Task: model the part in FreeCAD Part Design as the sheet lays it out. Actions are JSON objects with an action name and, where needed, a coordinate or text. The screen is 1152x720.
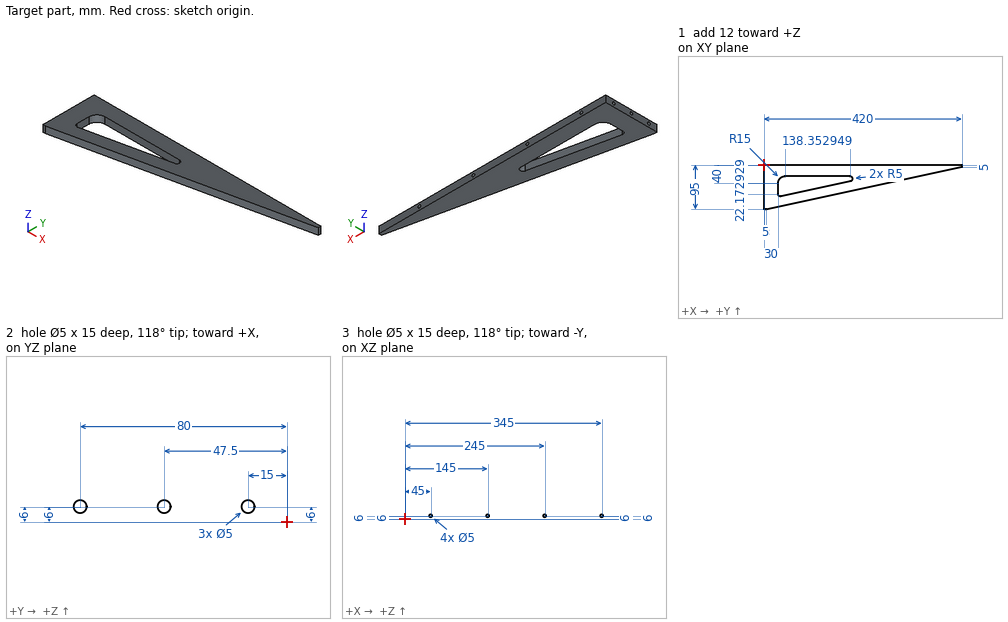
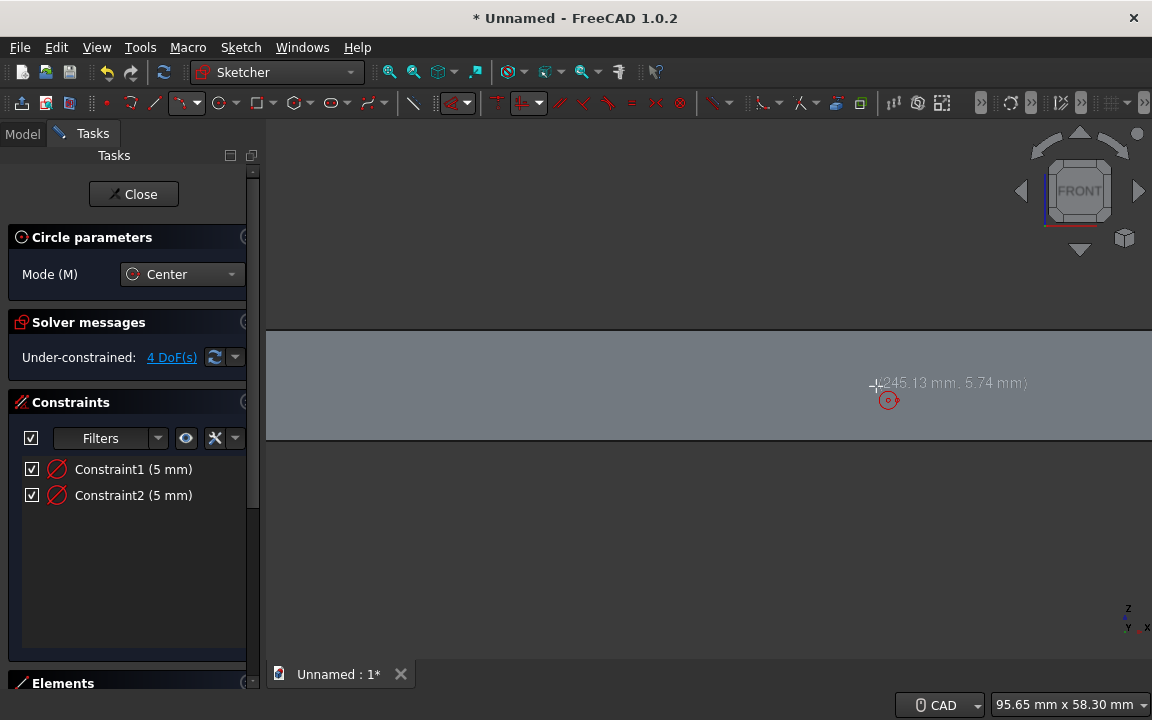
{"action": "scroll", "coordinate": [725, 386], "scroll_direction": "down", "scroll_amount": 9}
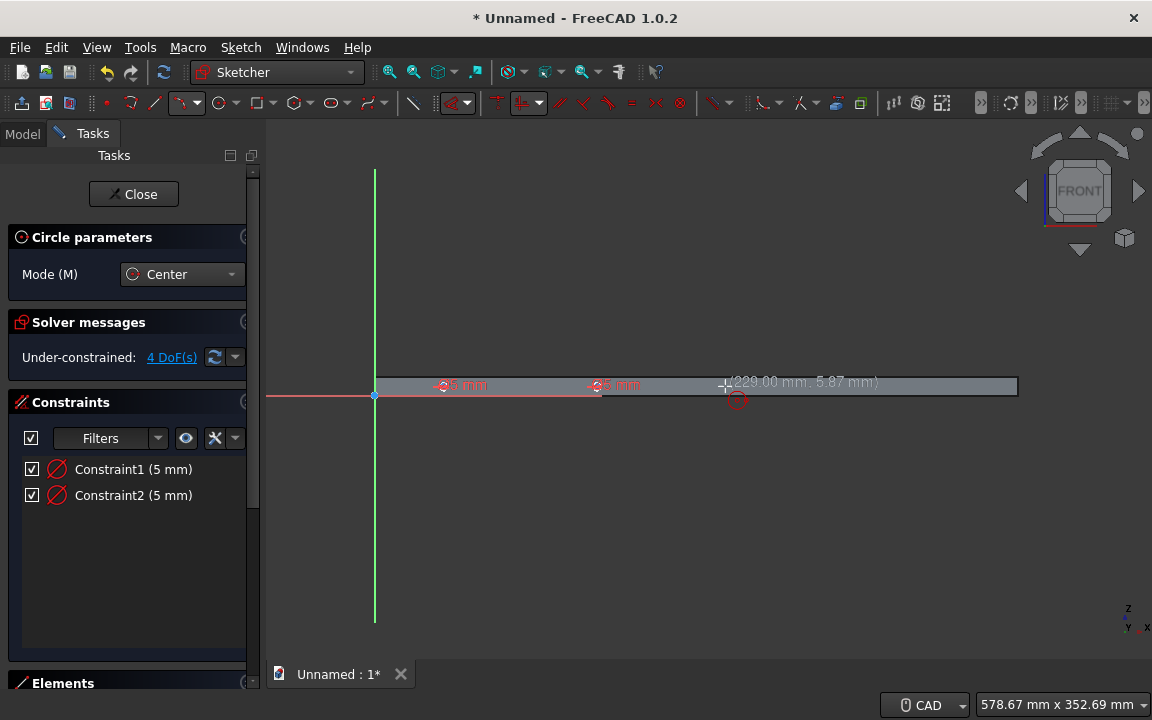
{"action": "scroll", "coordinate": [750, 386], "scroll_direction": "up", "scroll_amount": 3}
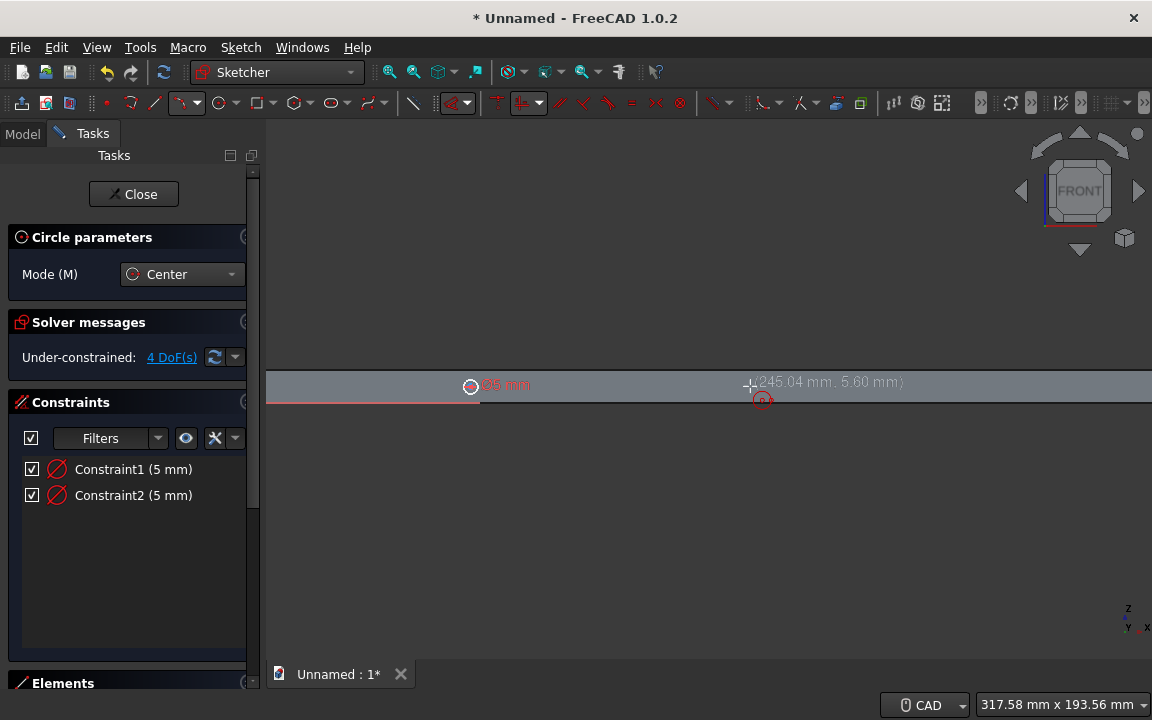
{"action": "left_click", "coordinate": [749, 386]}
{"action": "mouse_move", "coordinate": [754, 381]}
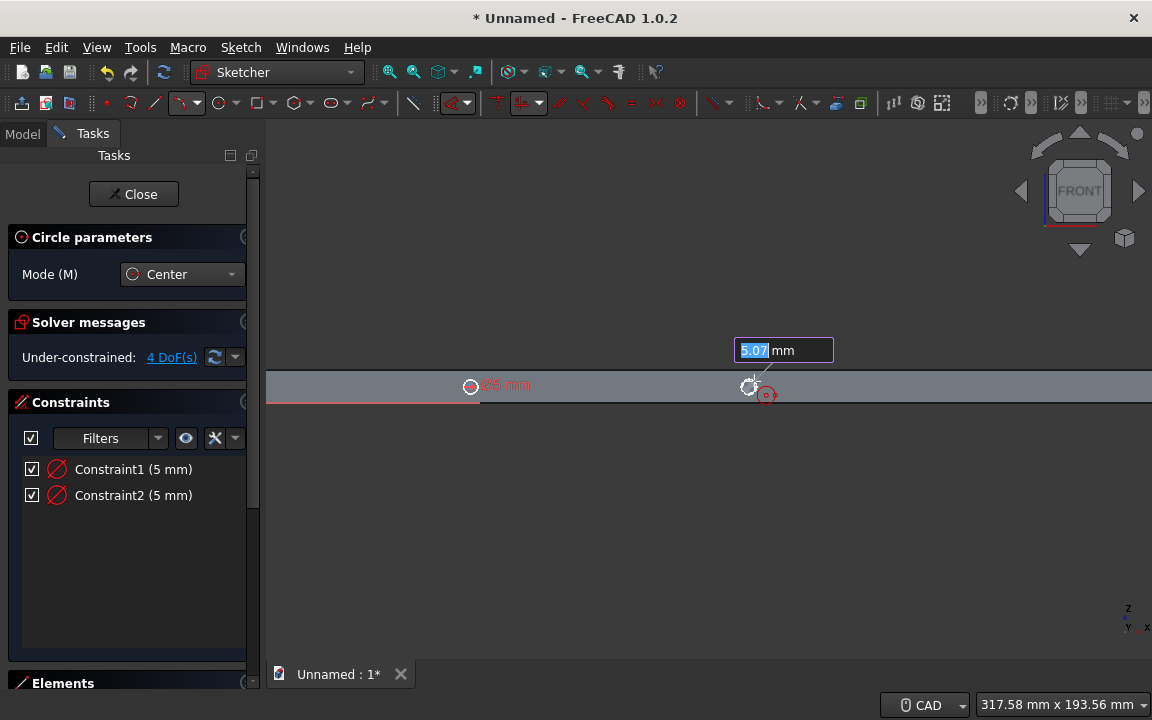
{"action": "type", "text": "5"}
{"action": "key", "text": "Return"}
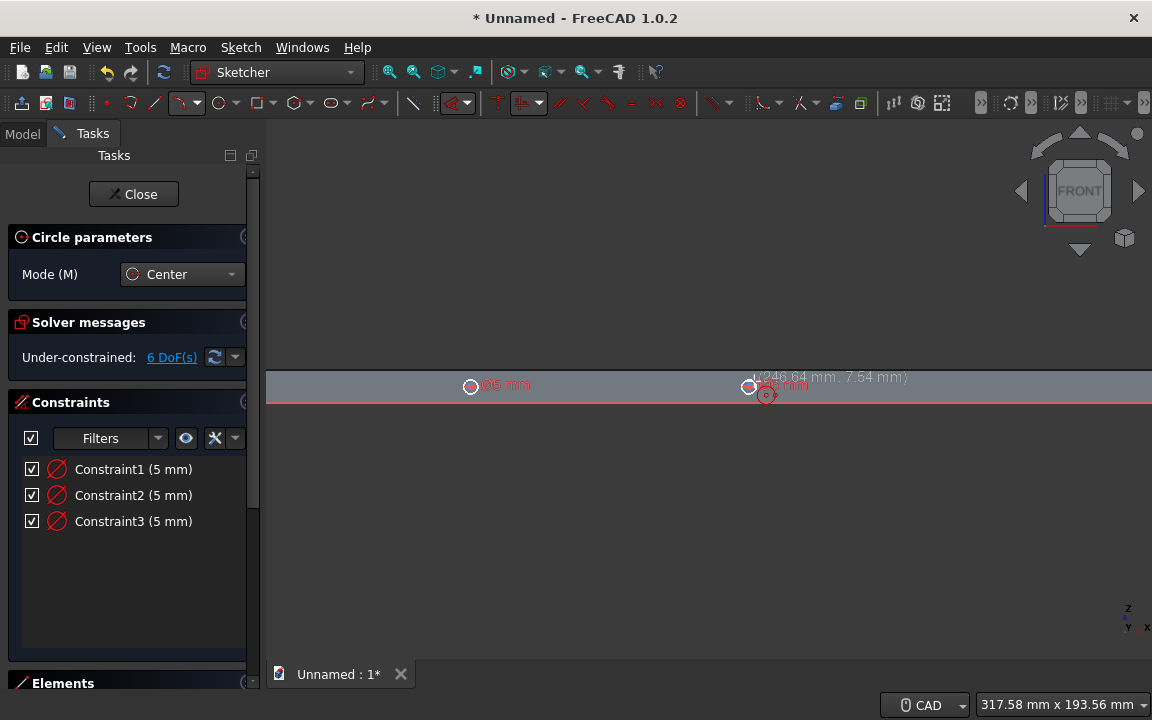
{"action": "scroll", "coordinate": [750, 386], "scroll_direction": "down", "scroll_amount": 3}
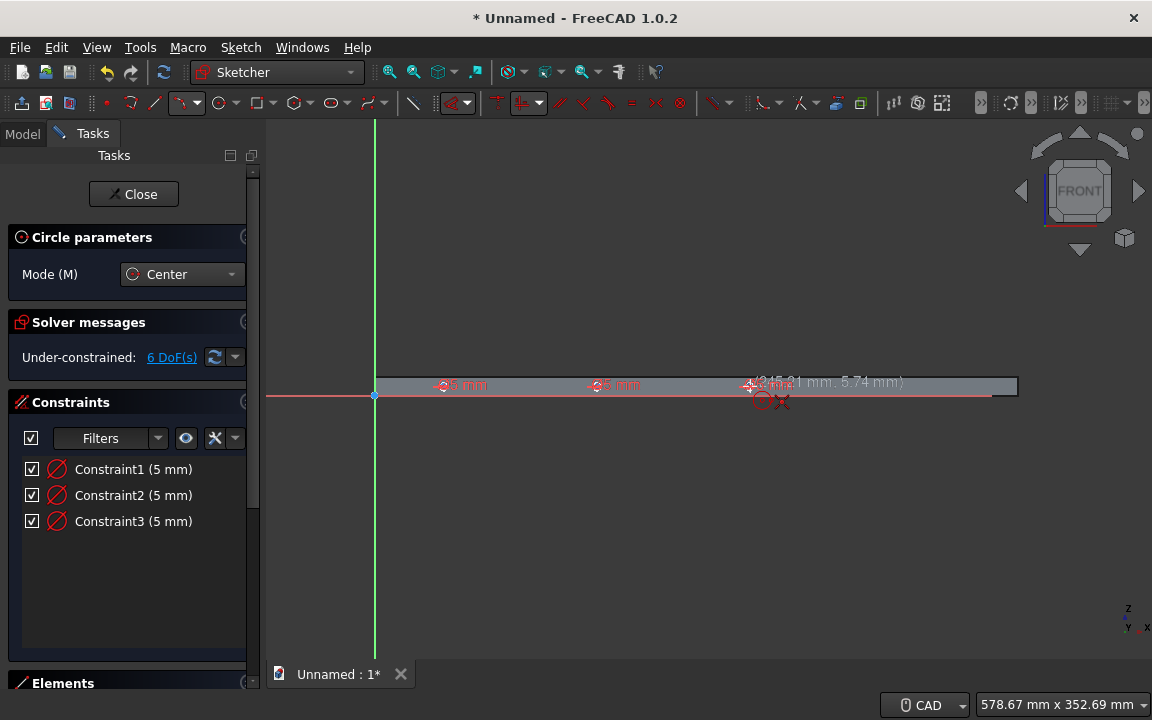
{"action": "scroll", "coordinate": [903, 386], "scroll_direction": "up", "scroll_amount": 9}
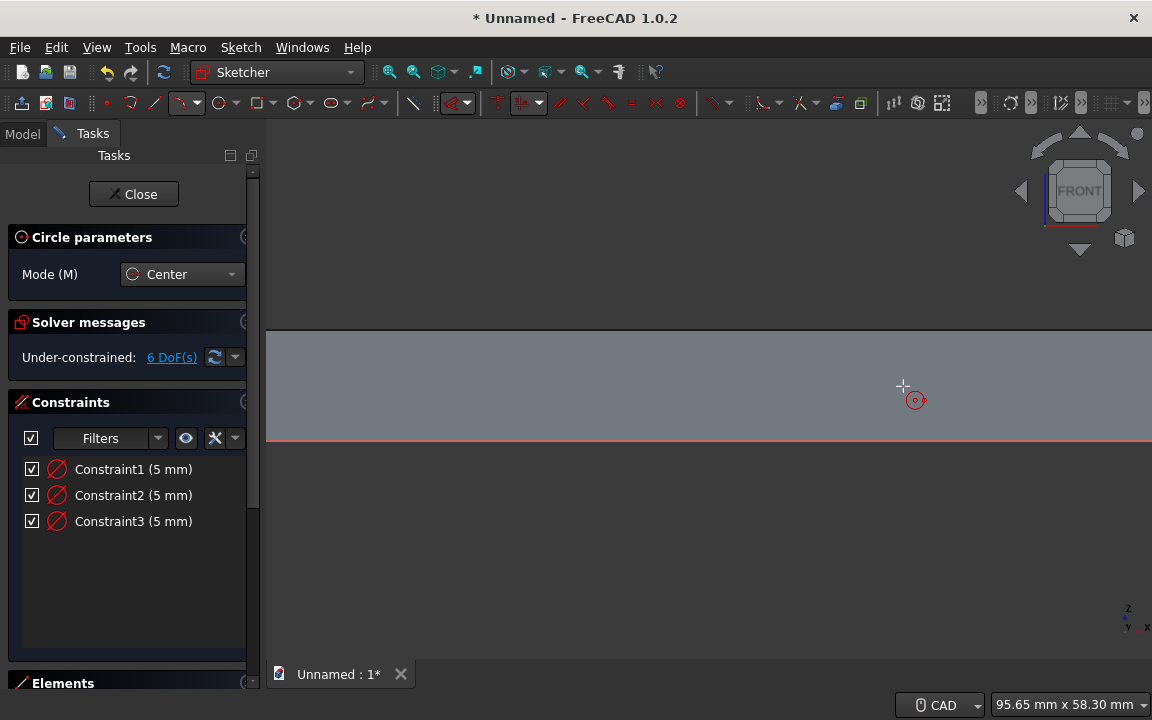
{"action": "scroll", "coordinate": [903, 386], "scroll_direction": "down", "scroll_amount": 9}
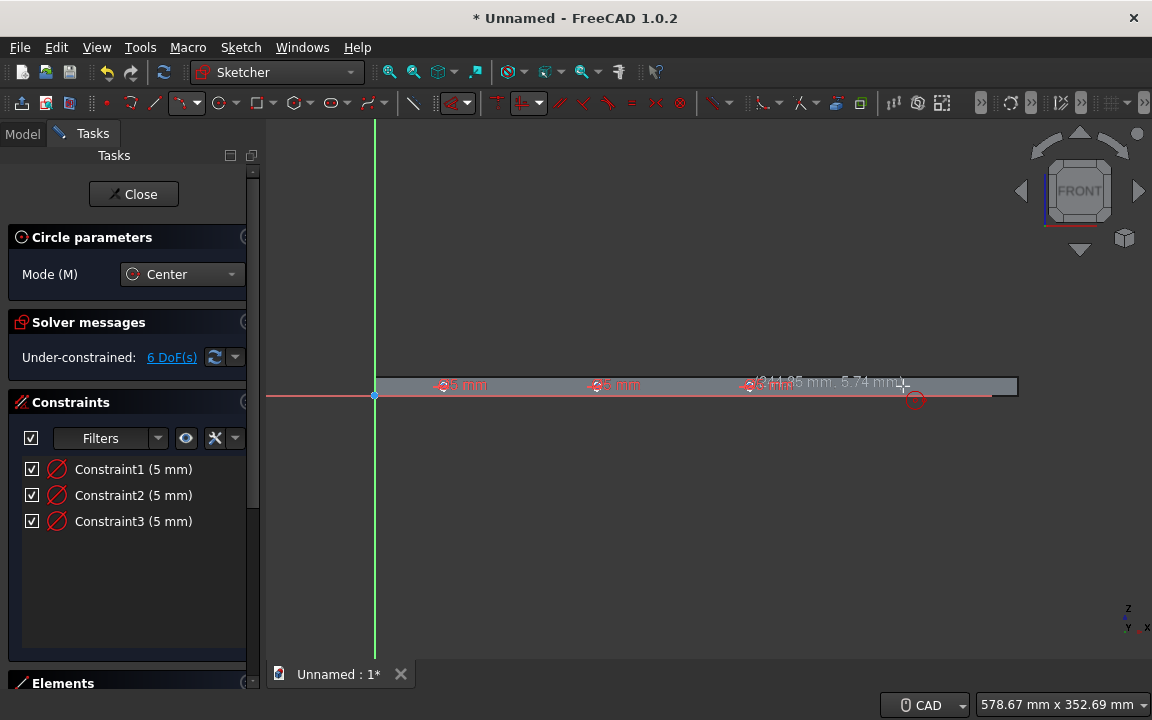
{"action": "scroll", "coordinate": [903, 386], "scroll_direction": "up", "scroll_amount": 3}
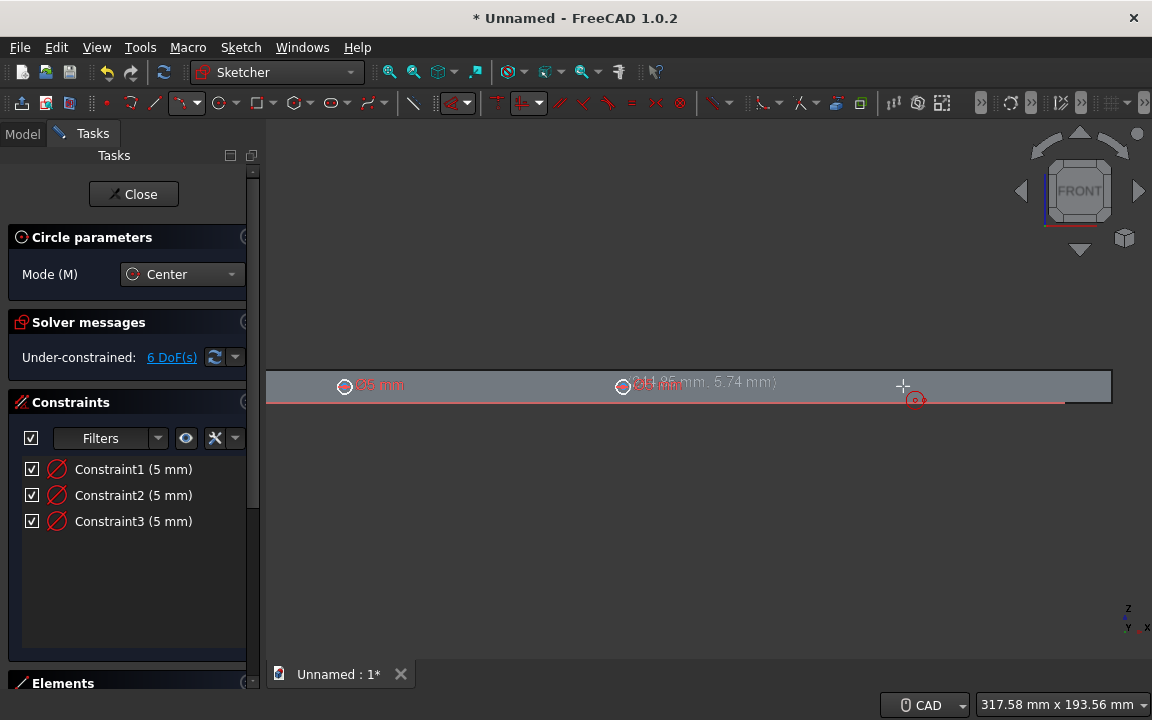
{"action": "left_click", "coordinate": [902, 386]}
{"action": "mouse_move", "coordinate": [907, 381]}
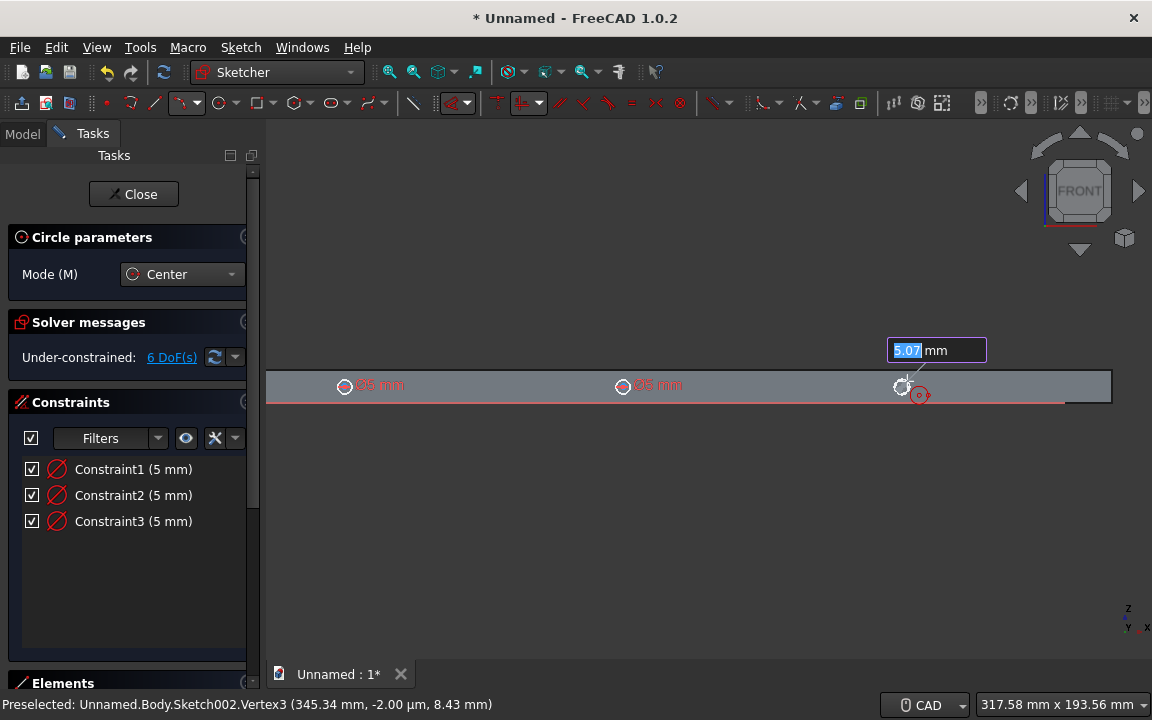
{"action": "type", "text": "5"}
{"action": "key", "text": "Return"}
{"action": "key", "text": "Escape"}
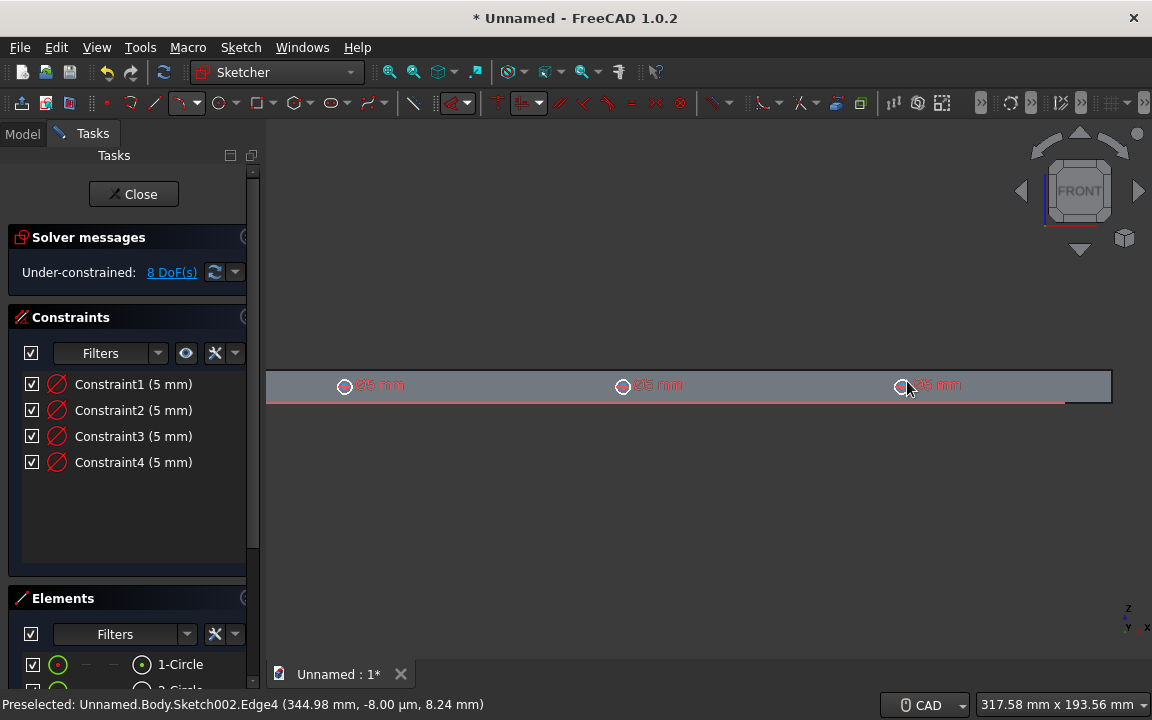
{"action": "scroll", "coordinate": [903, 386], "scroll_direction": "down", "scroll_amount": 3}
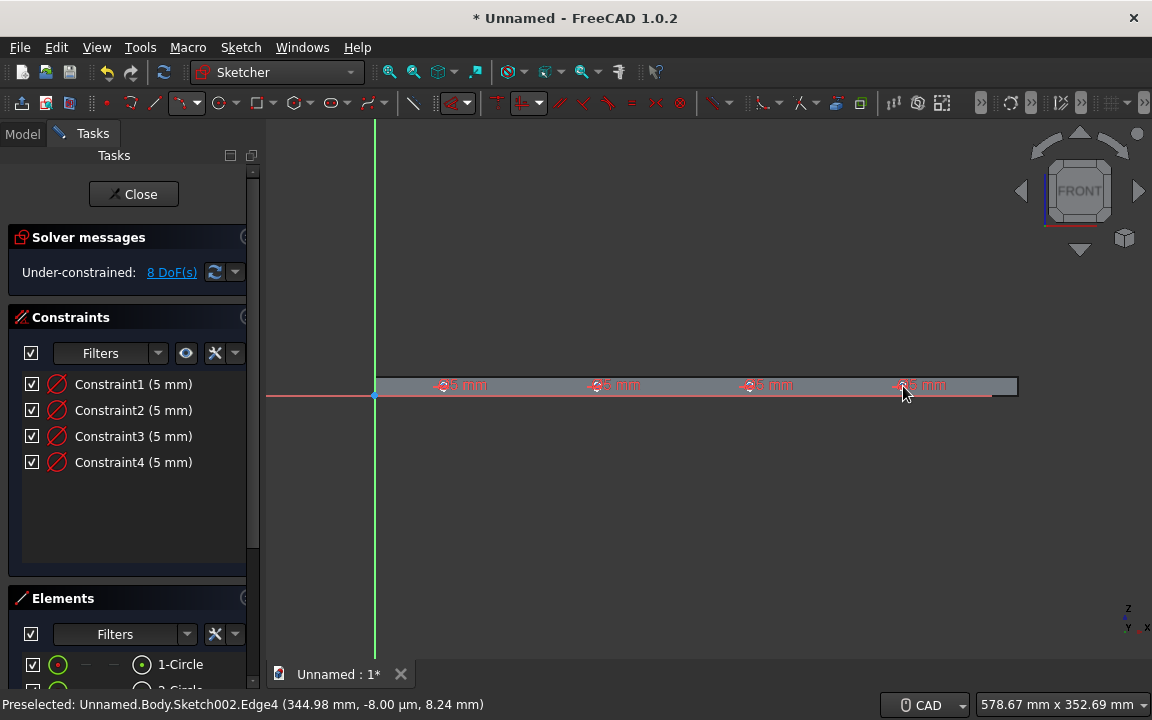
{"action": "scroll", "coordinate": [444, 387], "scroll_direction": "up", "scroll_amount": 8}